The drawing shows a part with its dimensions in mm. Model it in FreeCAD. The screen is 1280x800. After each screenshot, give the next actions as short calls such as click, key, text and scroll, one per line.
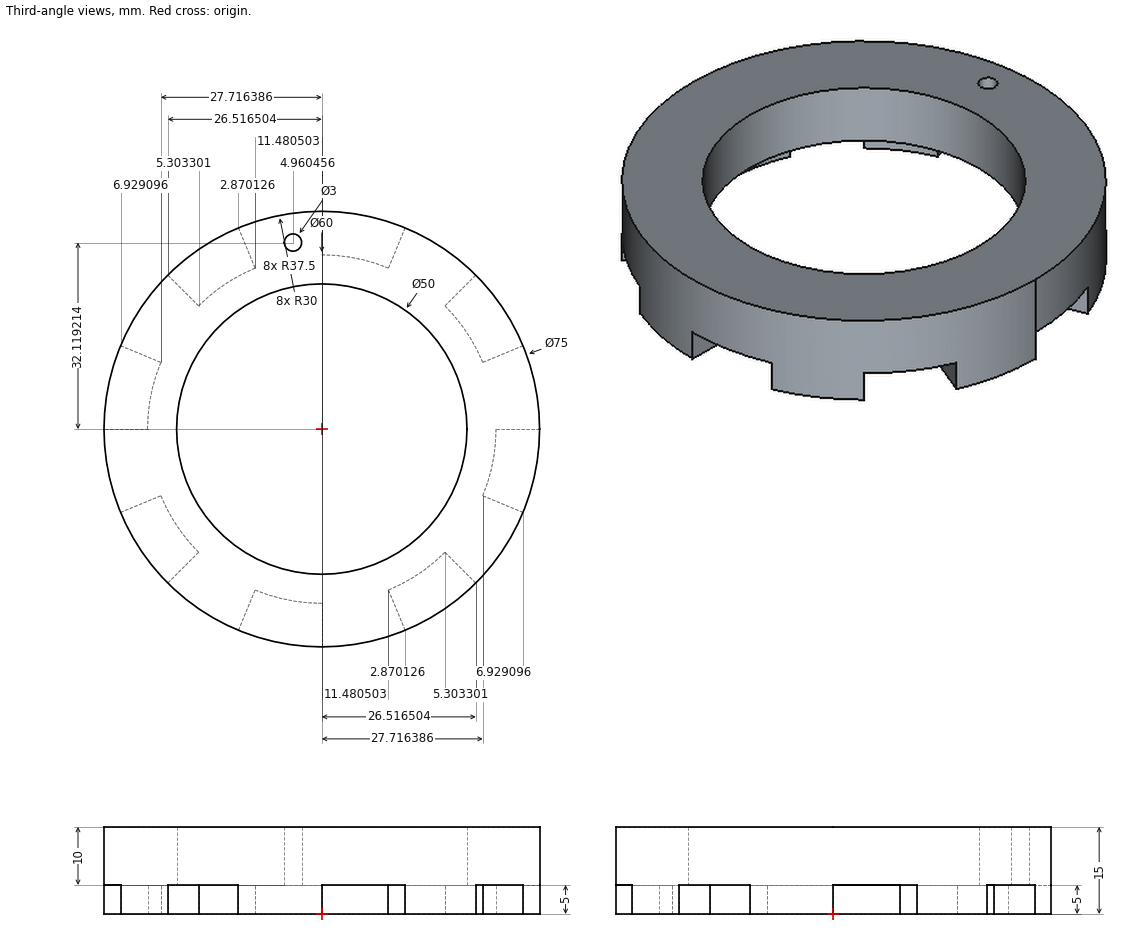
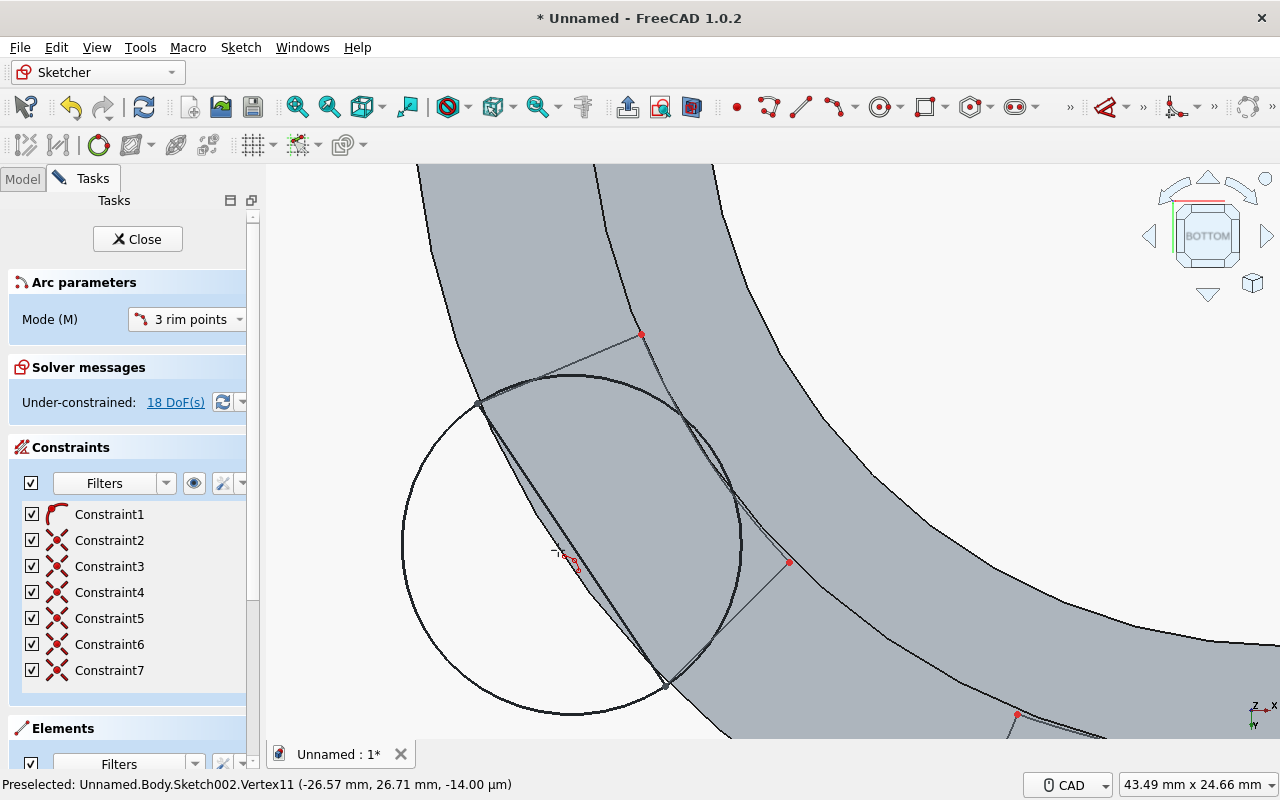
click(558, 549)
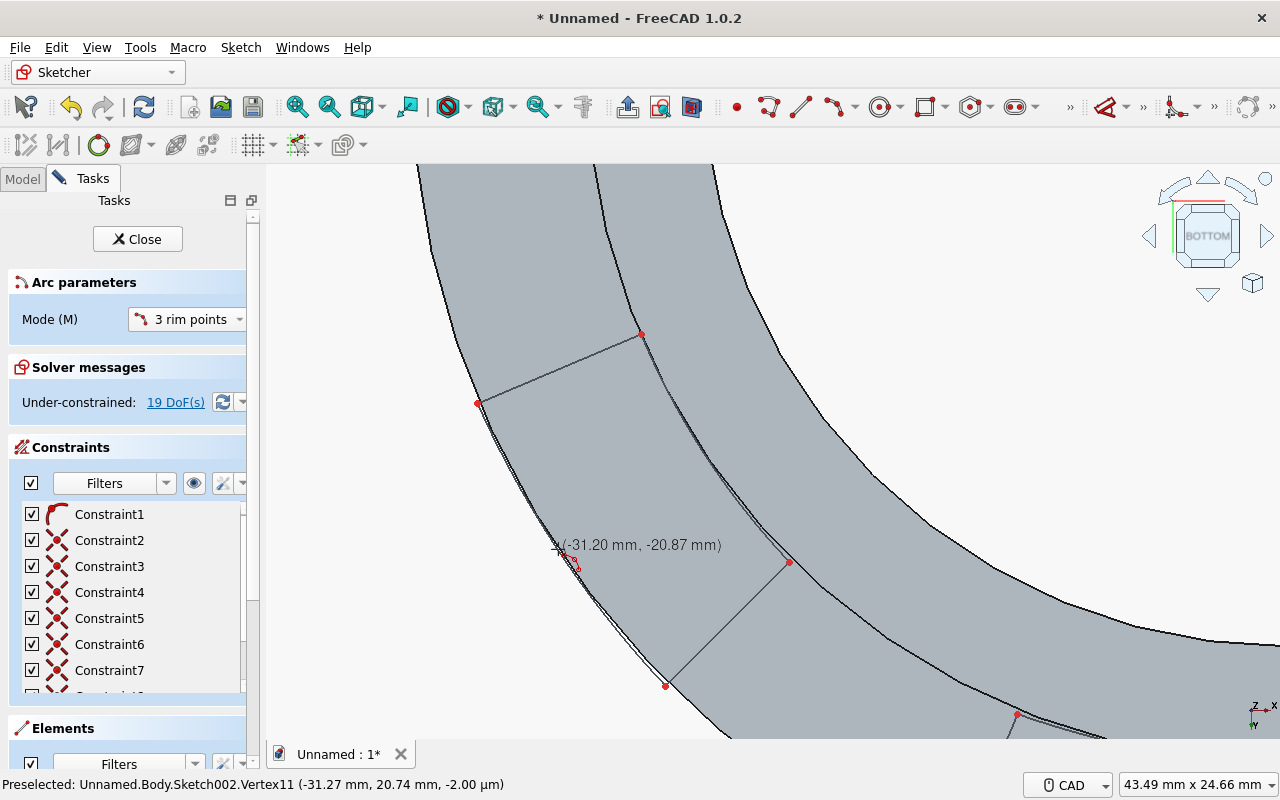
key(g)
key(l)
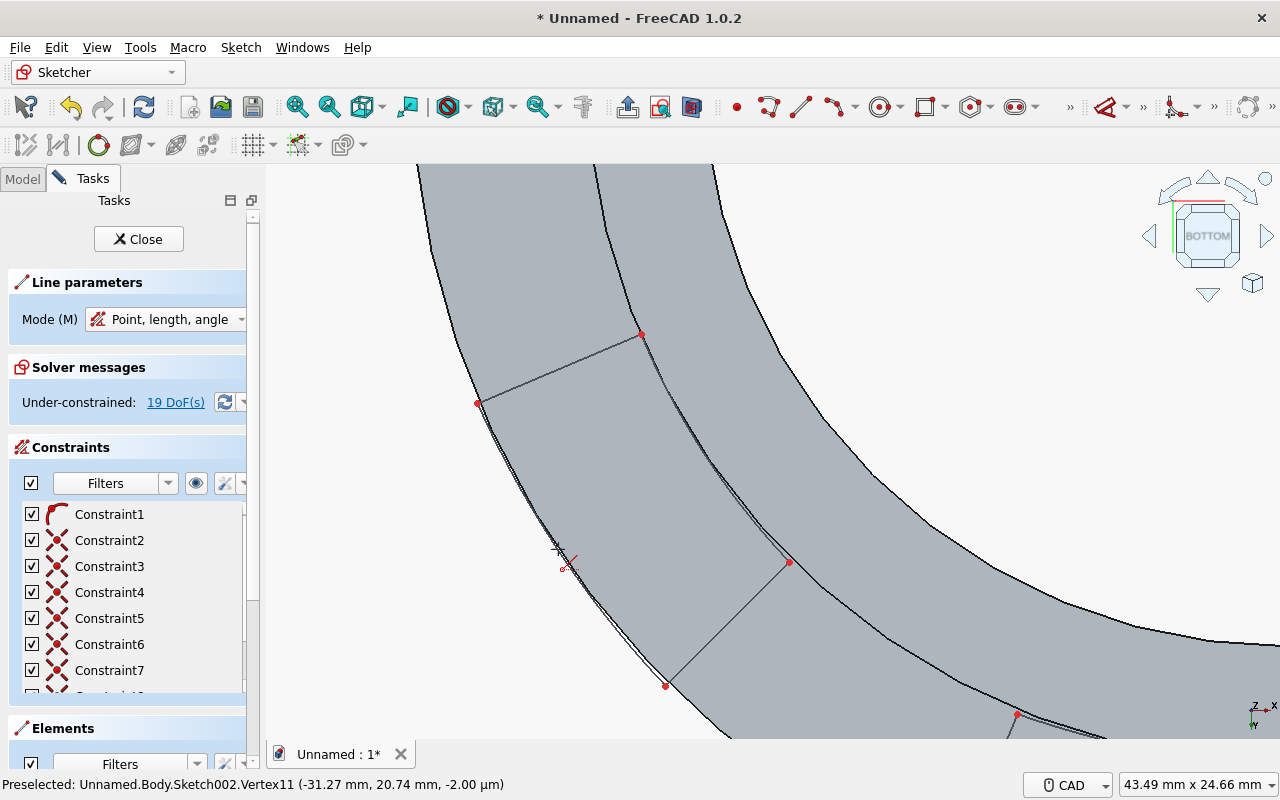
scroll(558, 550, down, 8)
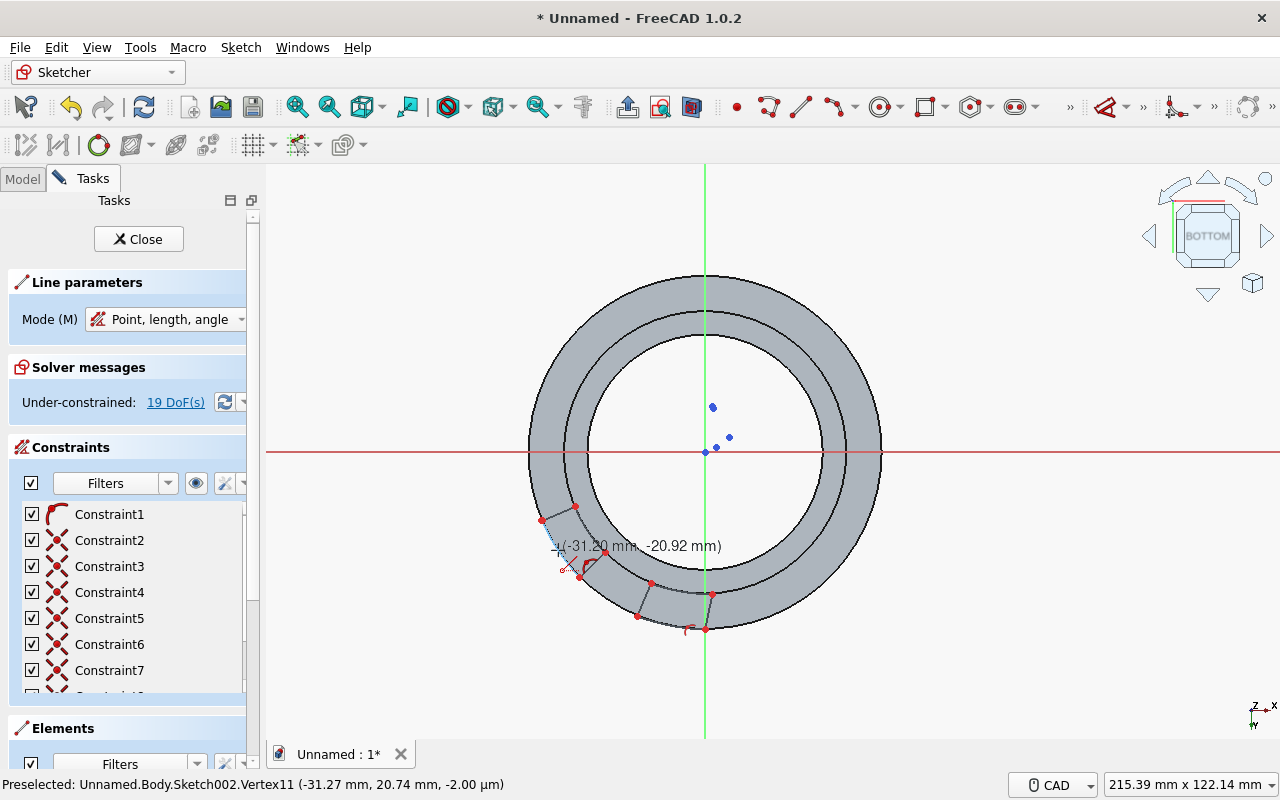
click(529, 452)
click(564, 443)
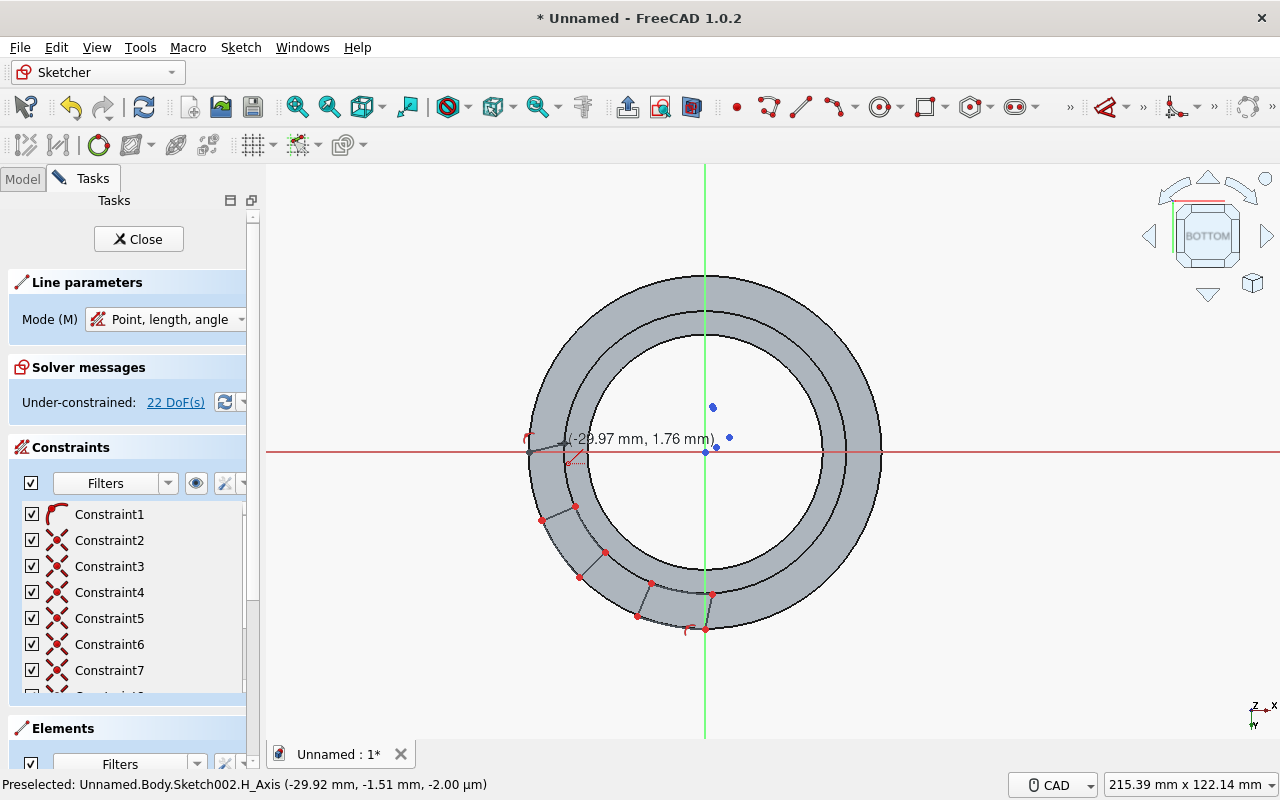
click(575, 398)
click(542, 385)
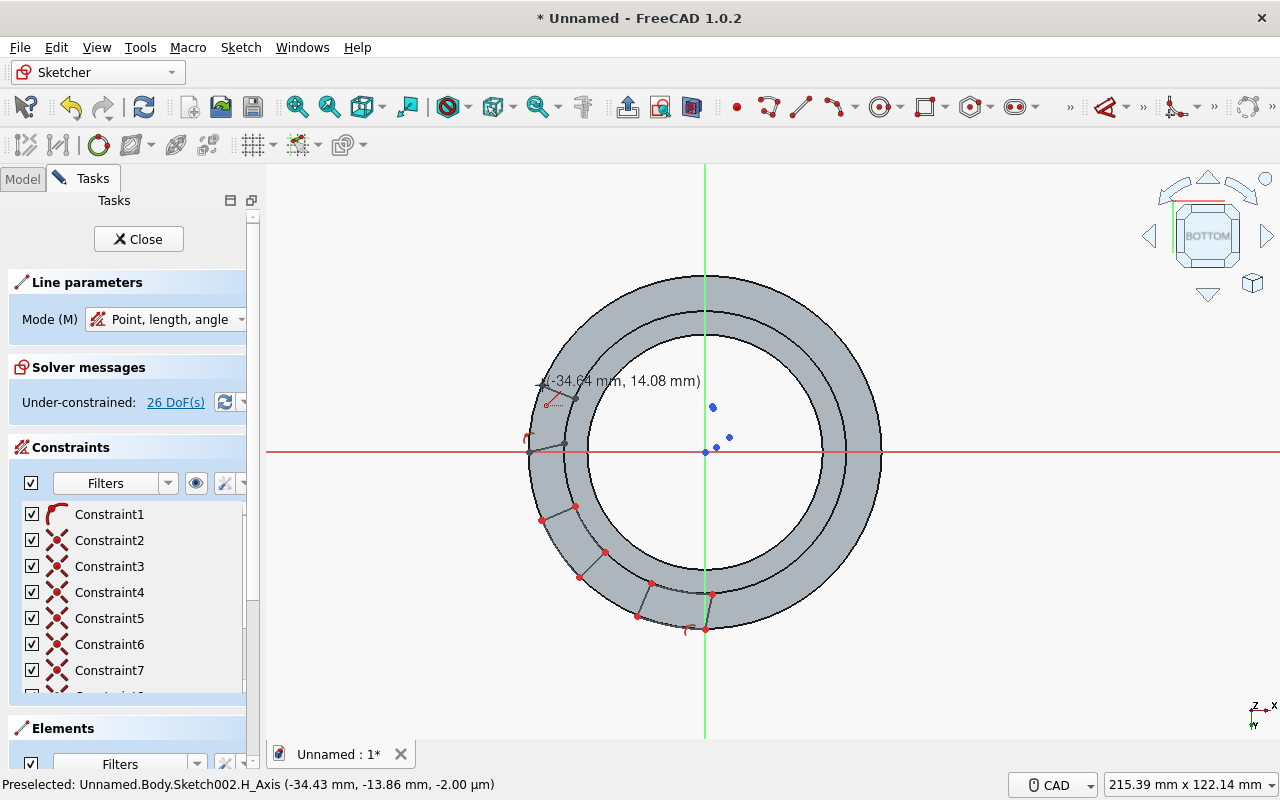
key(g)
key(3)
key(a)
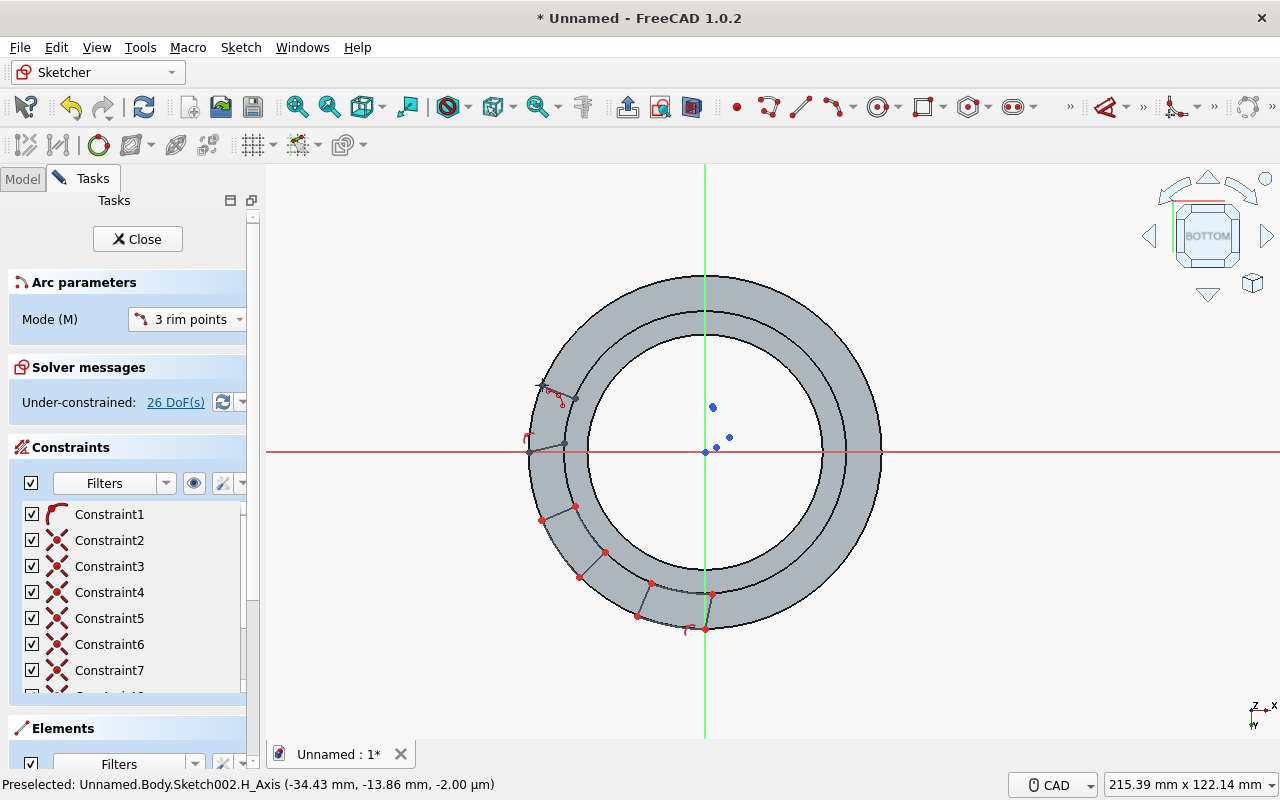
click(564, 444)
click(575, 399)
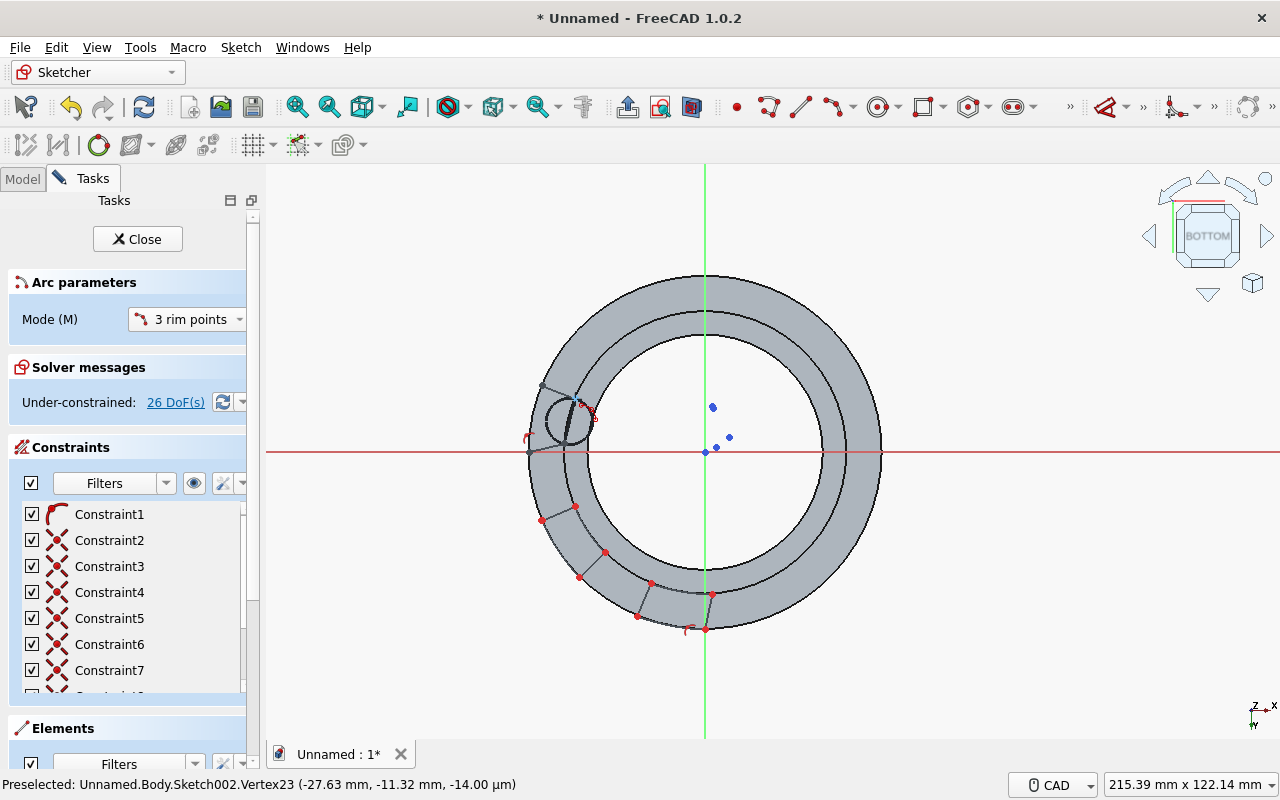
scroll(567, 425, up, 9)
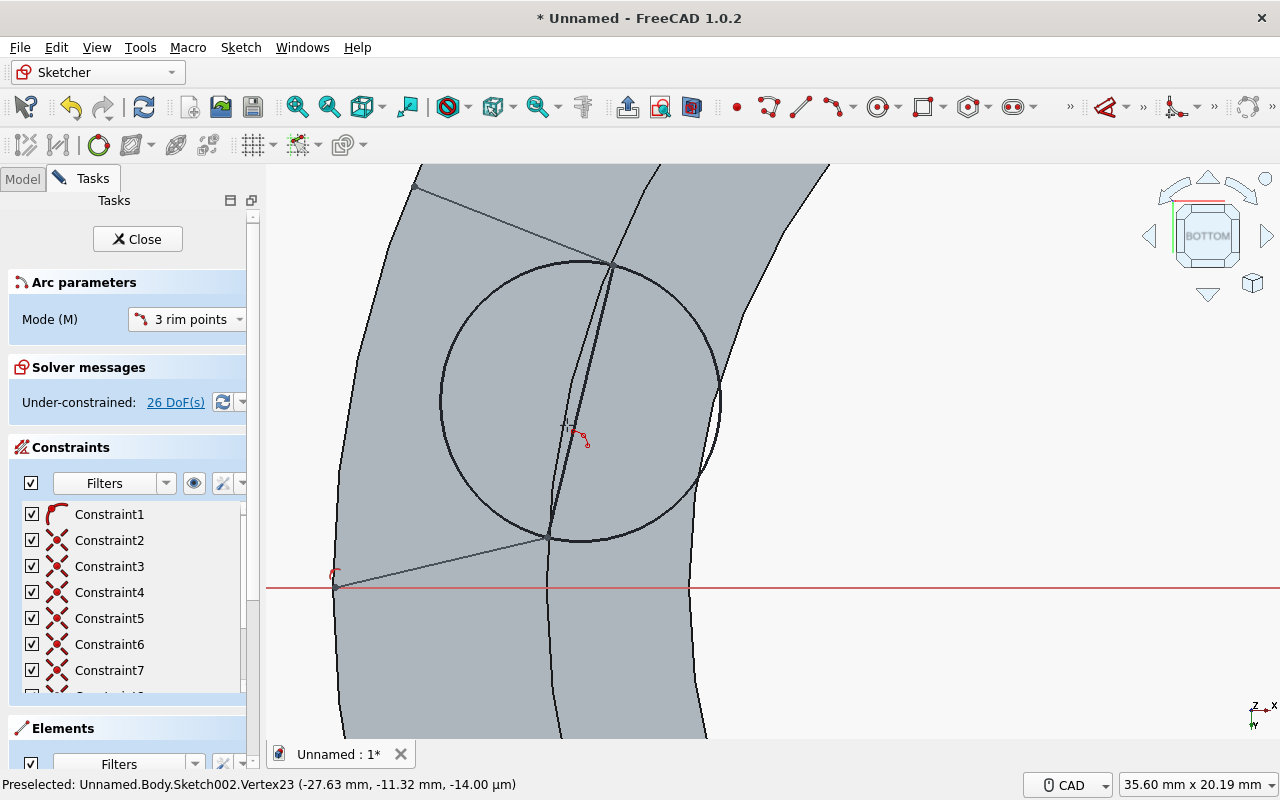
click(563, 421)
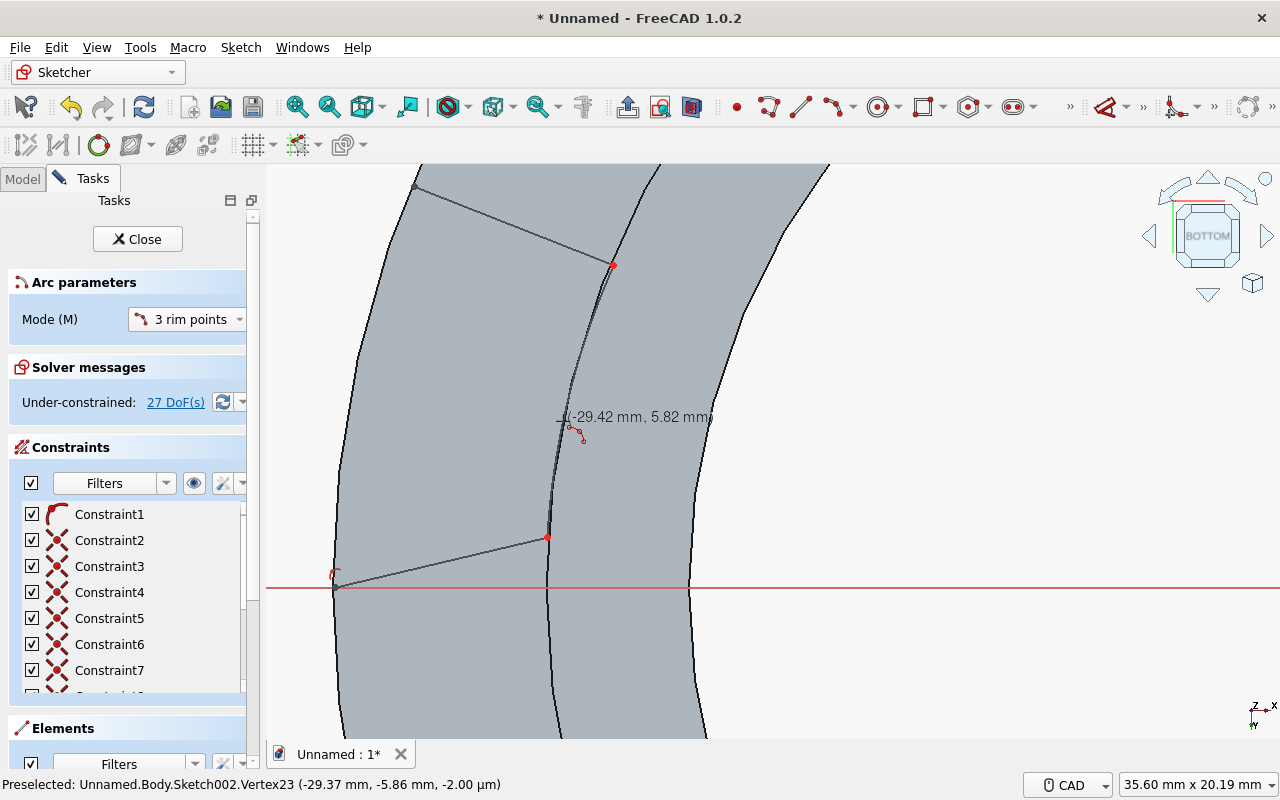
scroll(567, 425, down, 9)